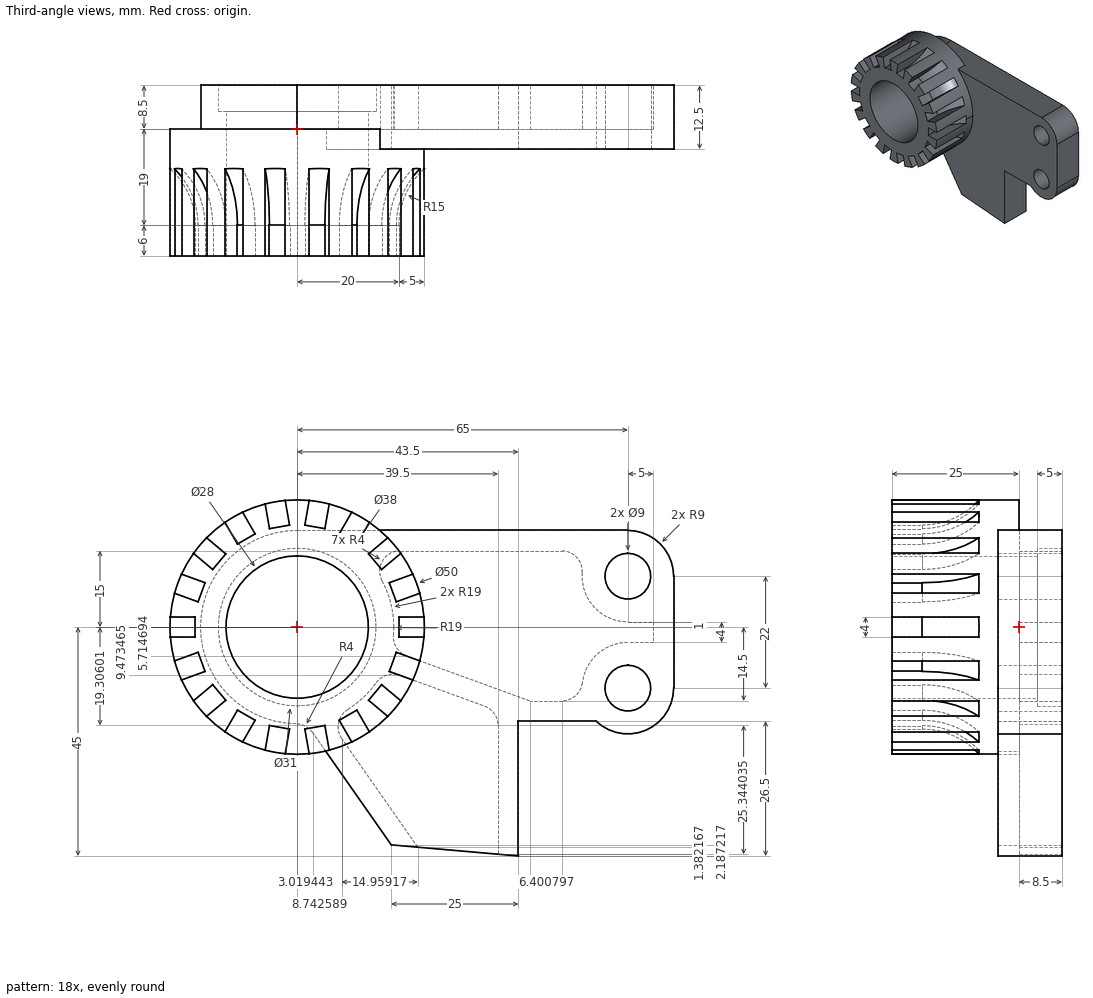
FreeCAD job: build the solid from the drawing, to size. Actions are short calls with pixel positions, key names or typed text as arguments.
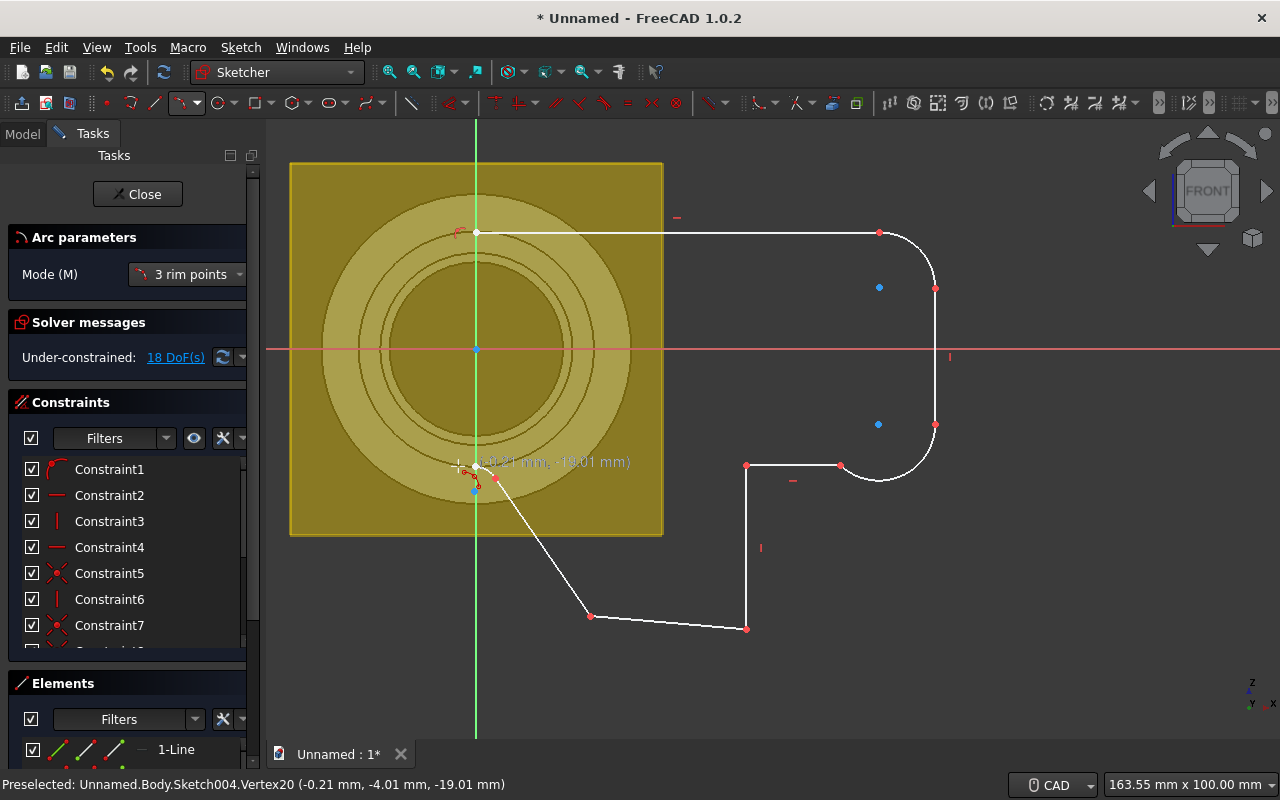
click(476, 233)
click(588, 386)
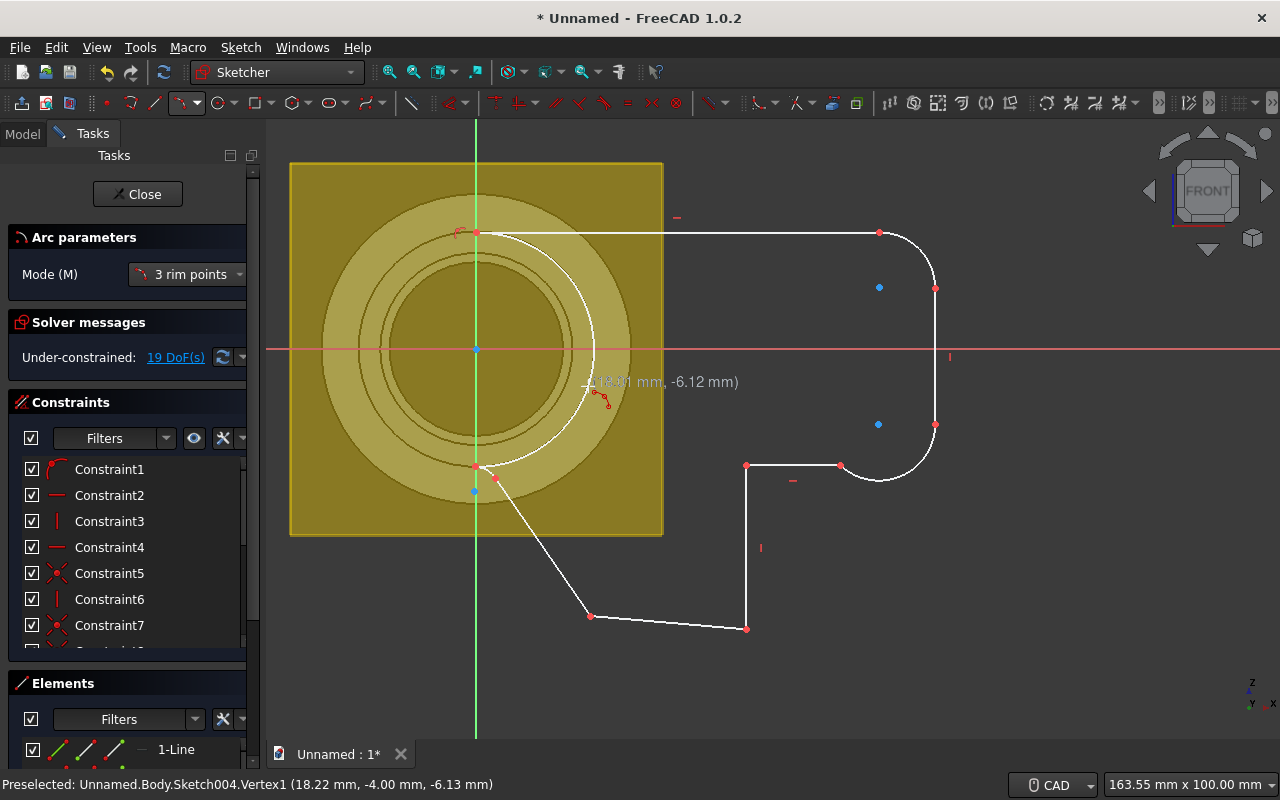
click(218, 104)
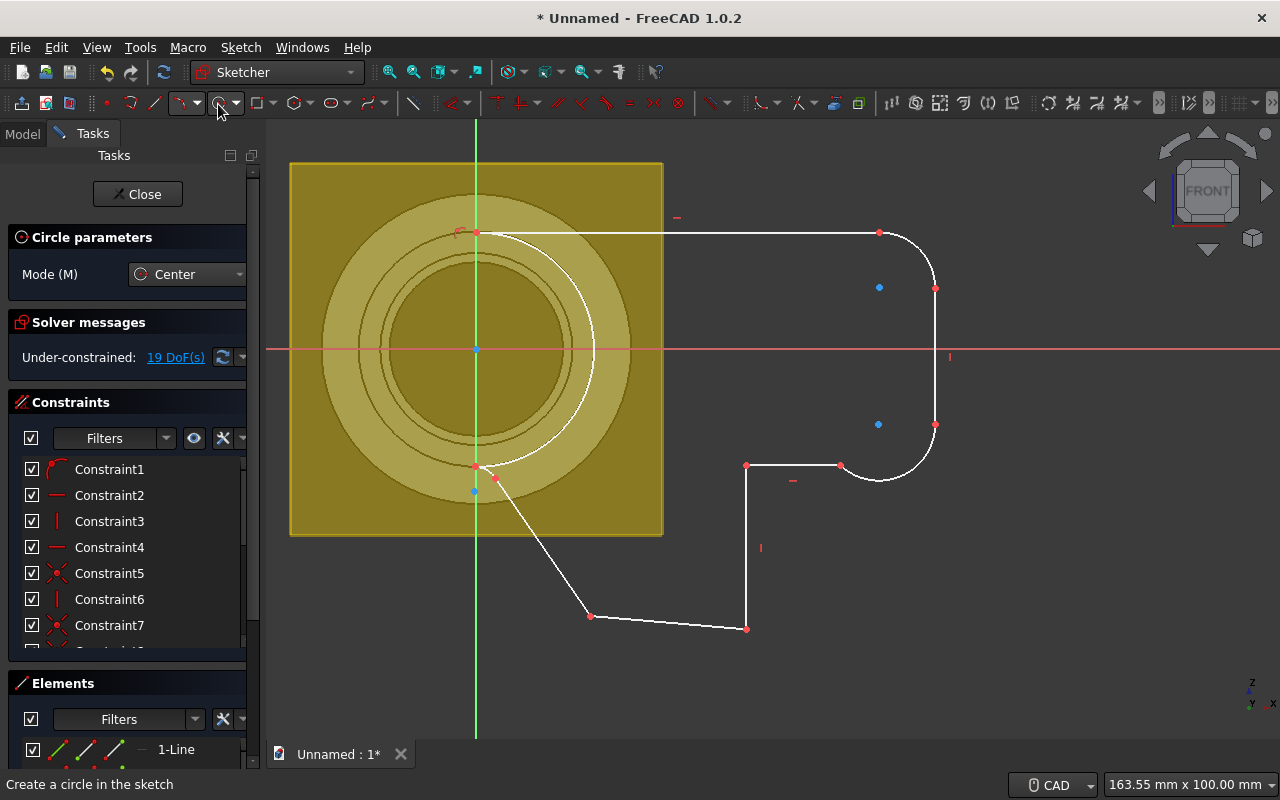
click(879, 287)
move(899, 267)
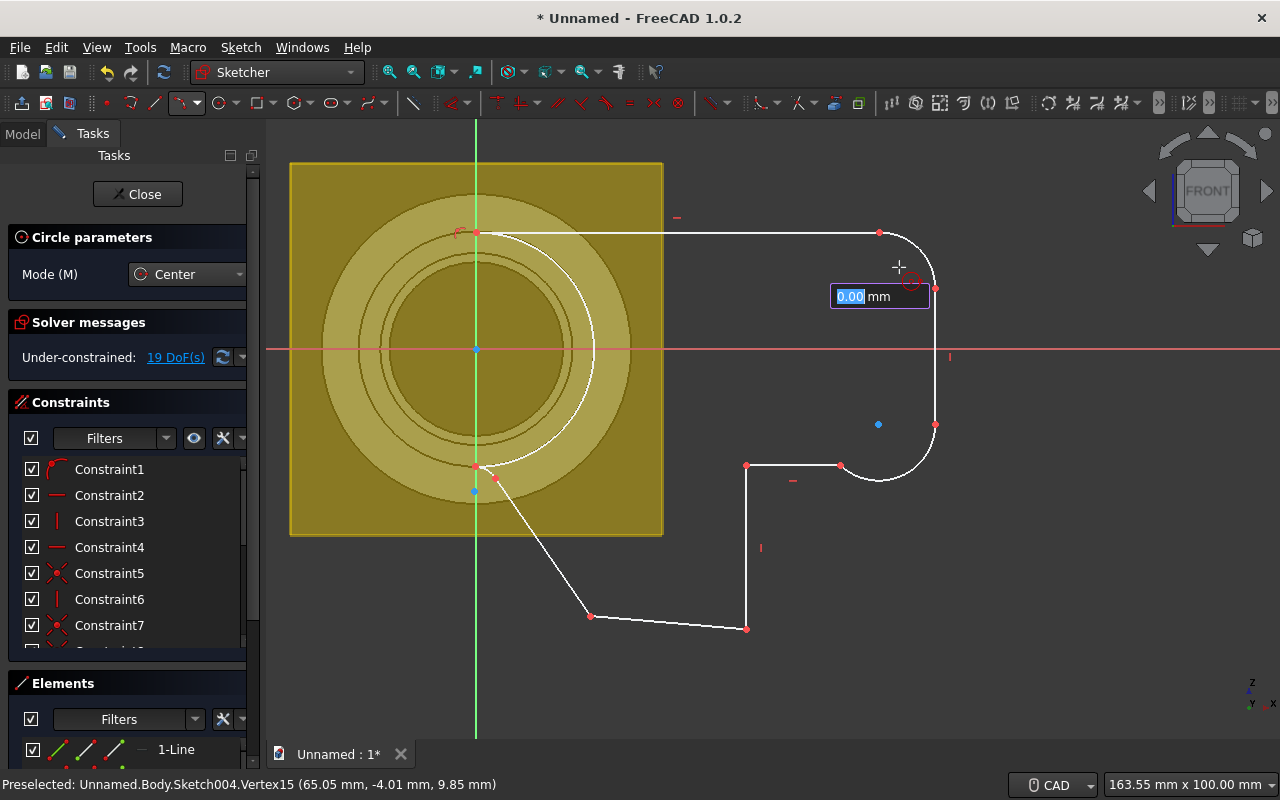
text(9)
key(Return)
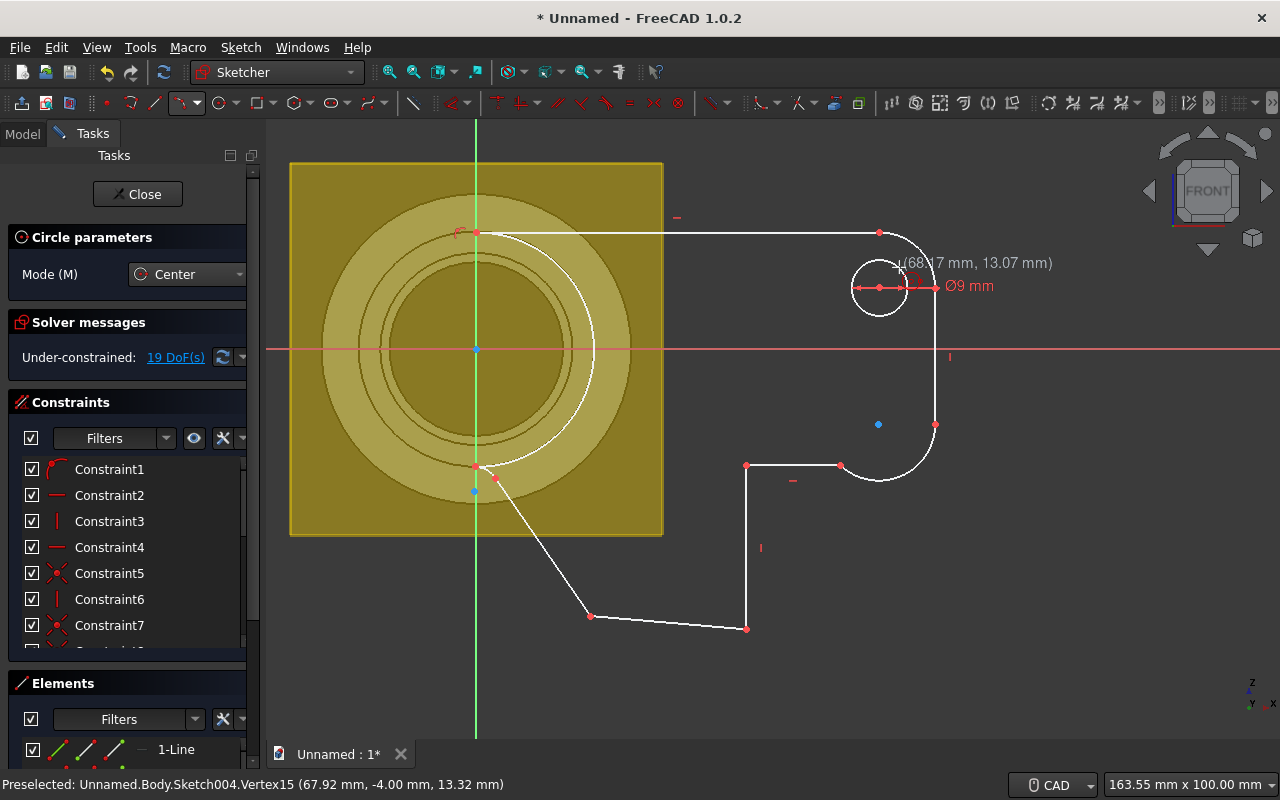
click(879, 423)
move(899, 404)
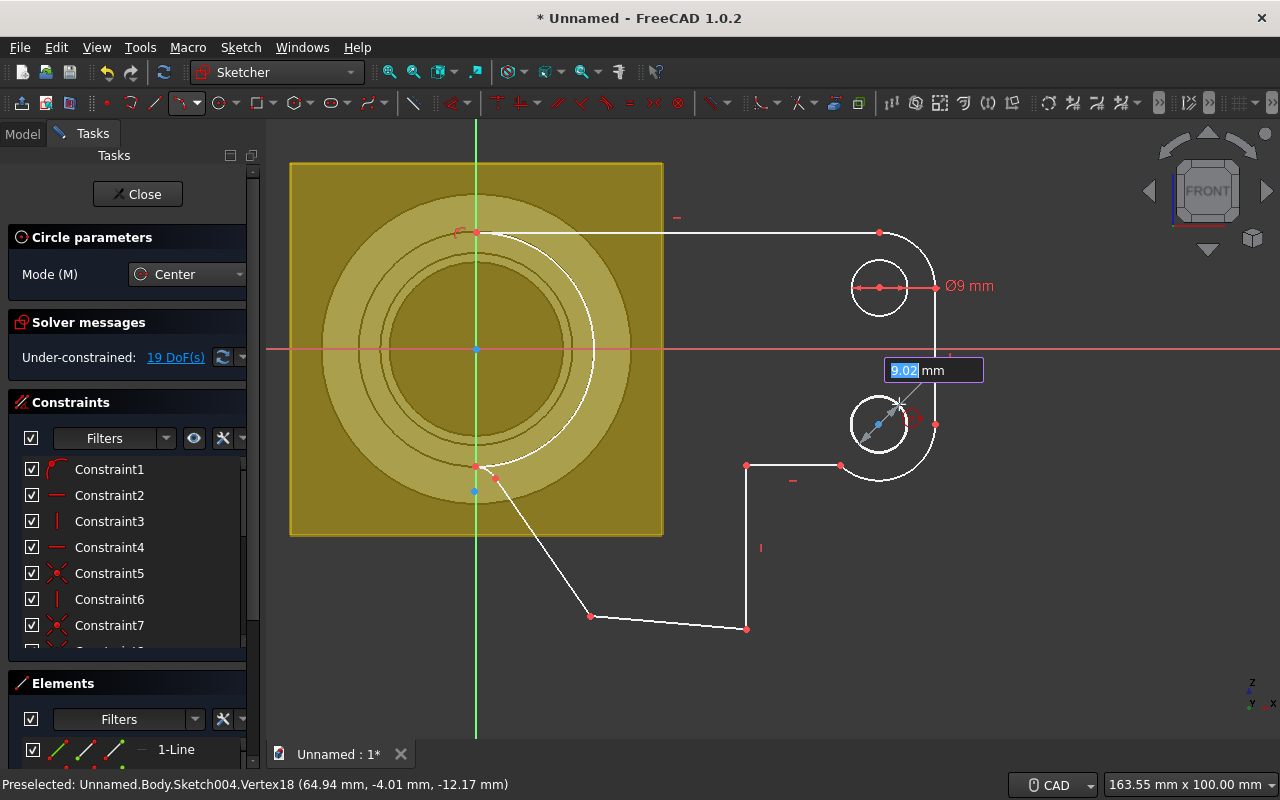
text(9)
key(Return)
key(Escape)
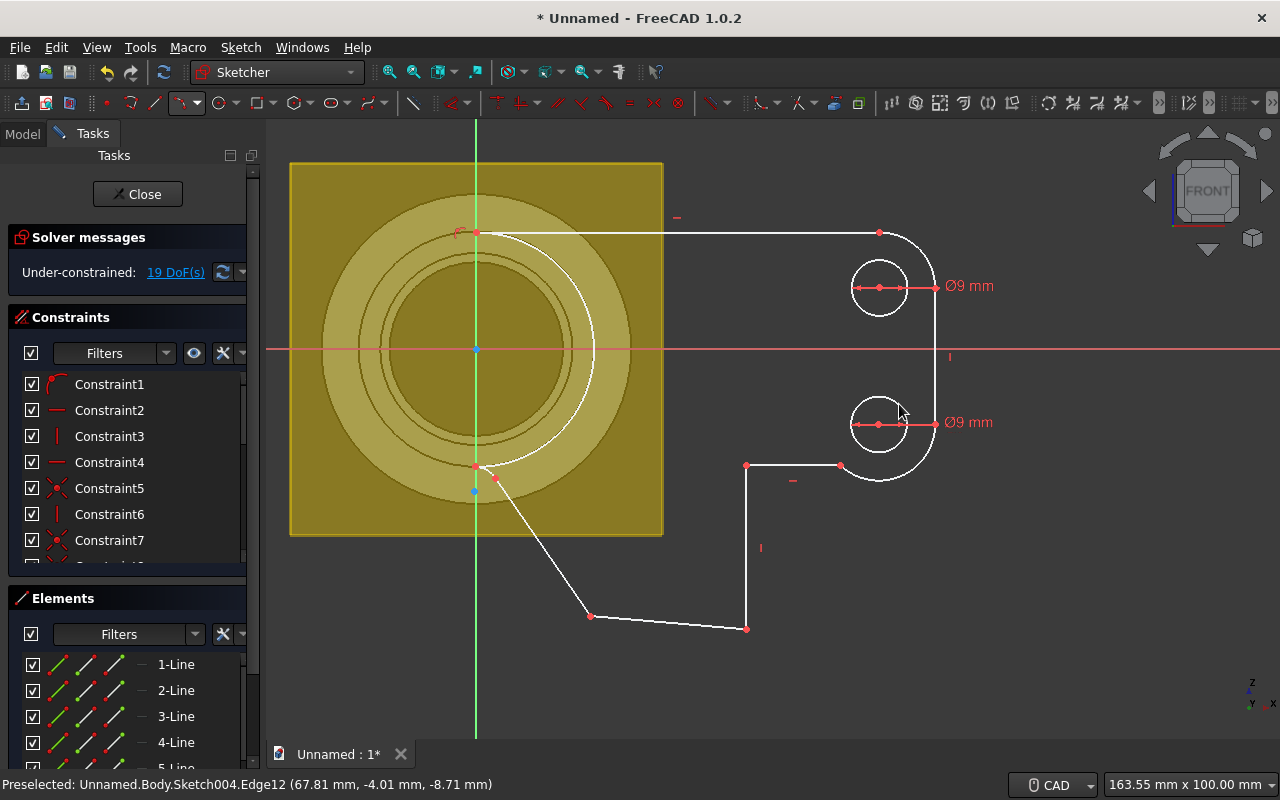
click(597, 233)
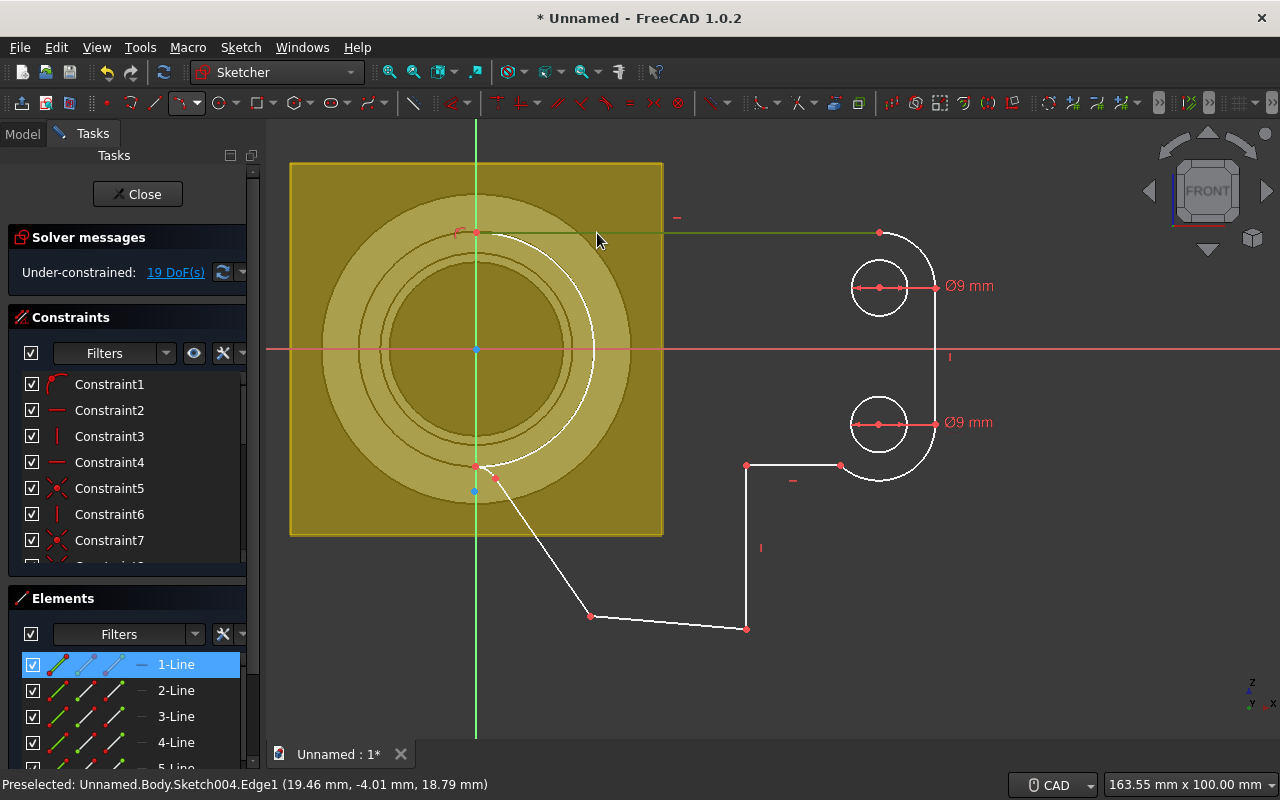
click(929, 263)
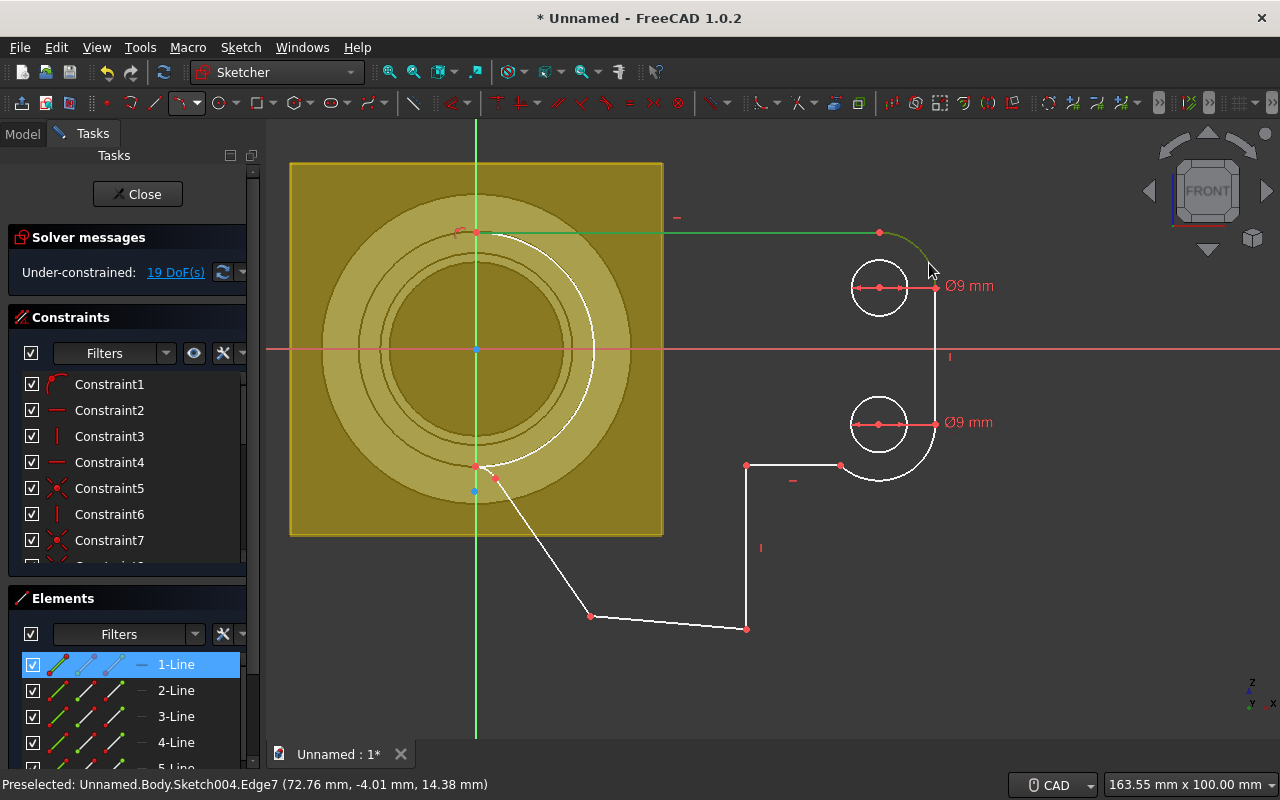
click(606, 104)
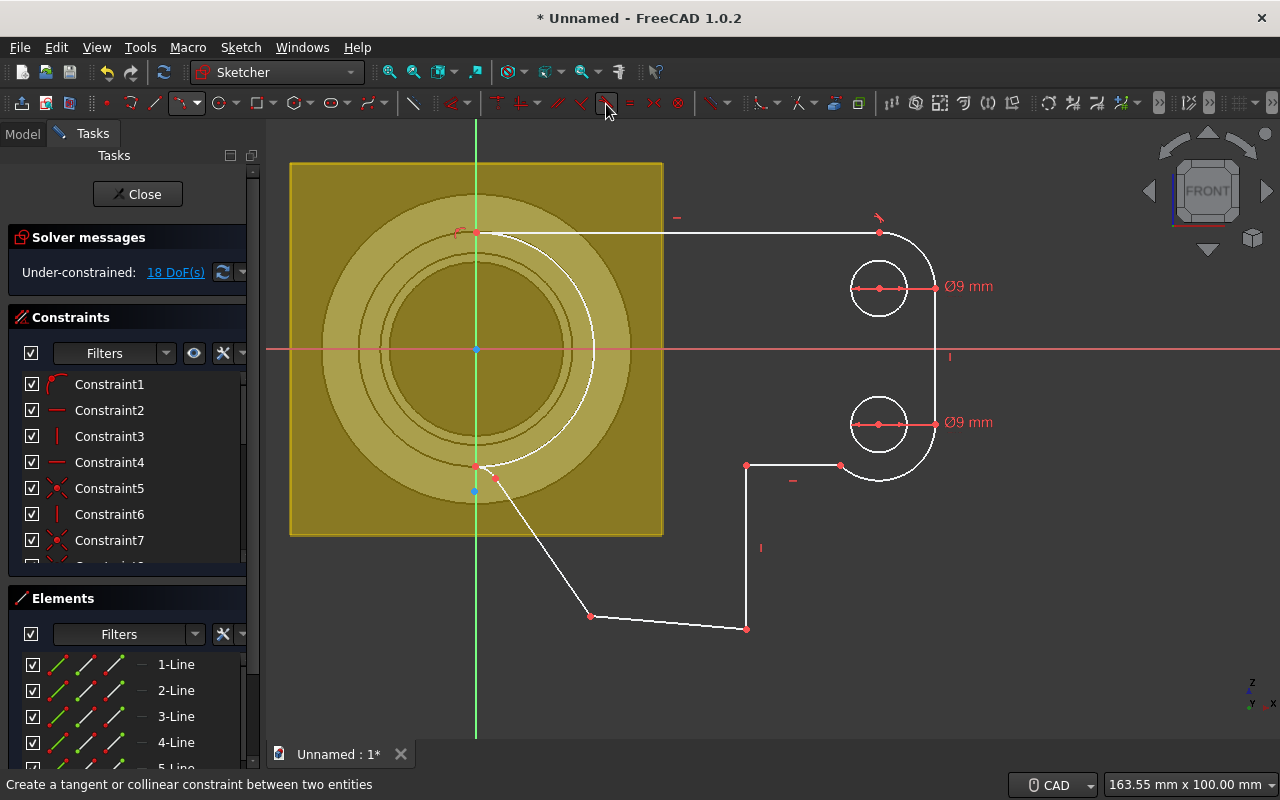
click(597, 233)